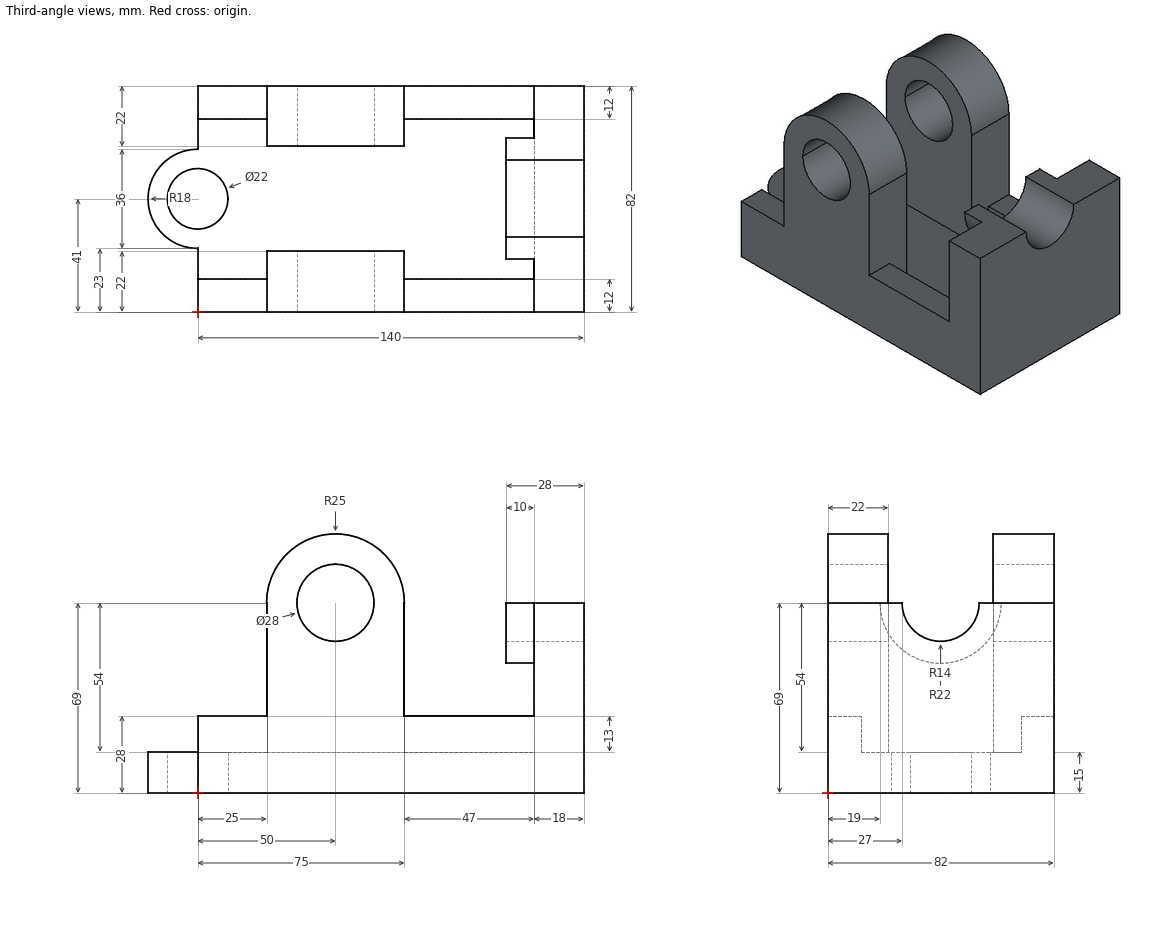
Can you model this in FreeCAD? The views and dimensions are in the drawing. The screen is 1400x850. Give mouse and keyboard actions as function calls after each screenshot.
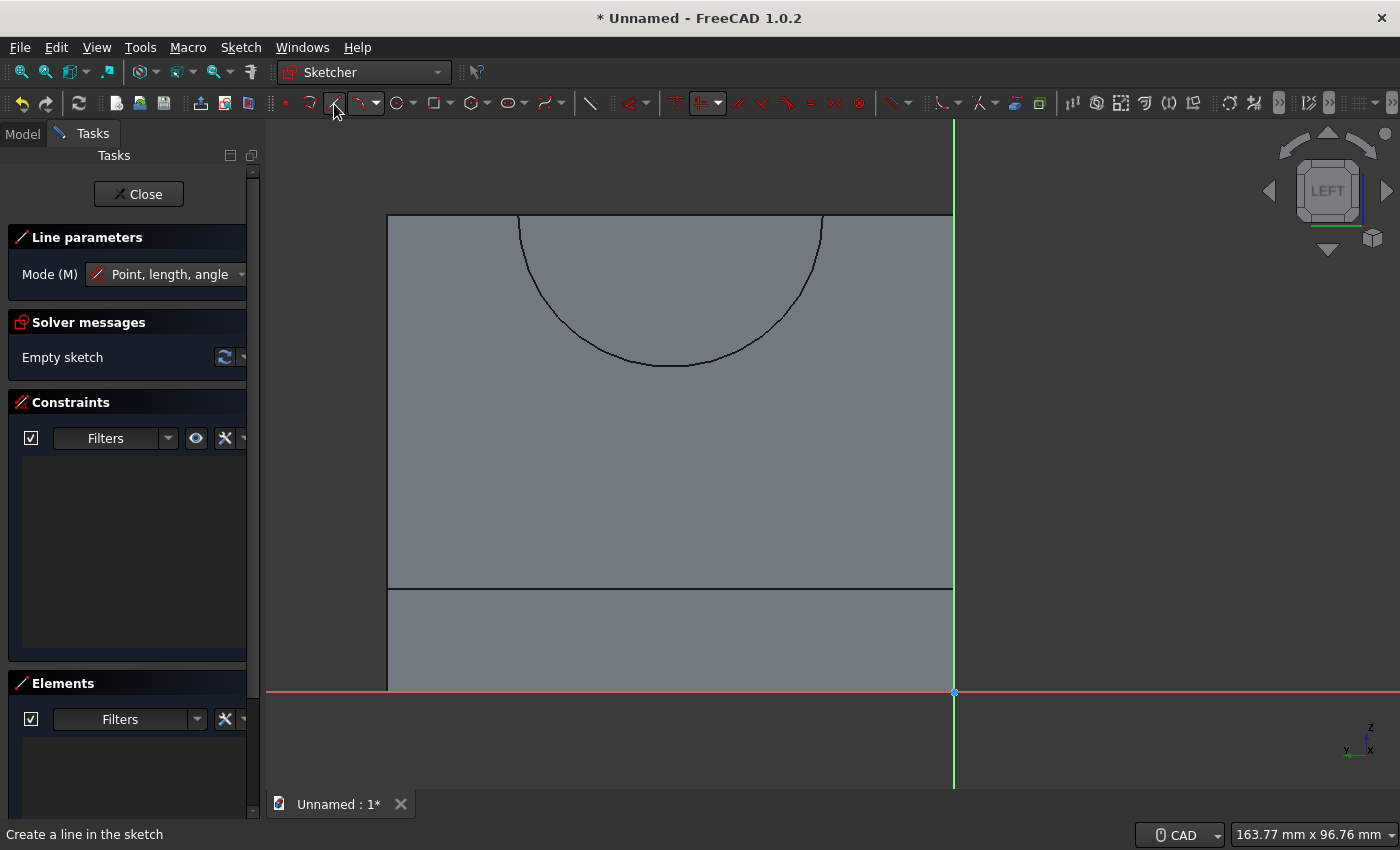
click(767, 215)
click(574, 215)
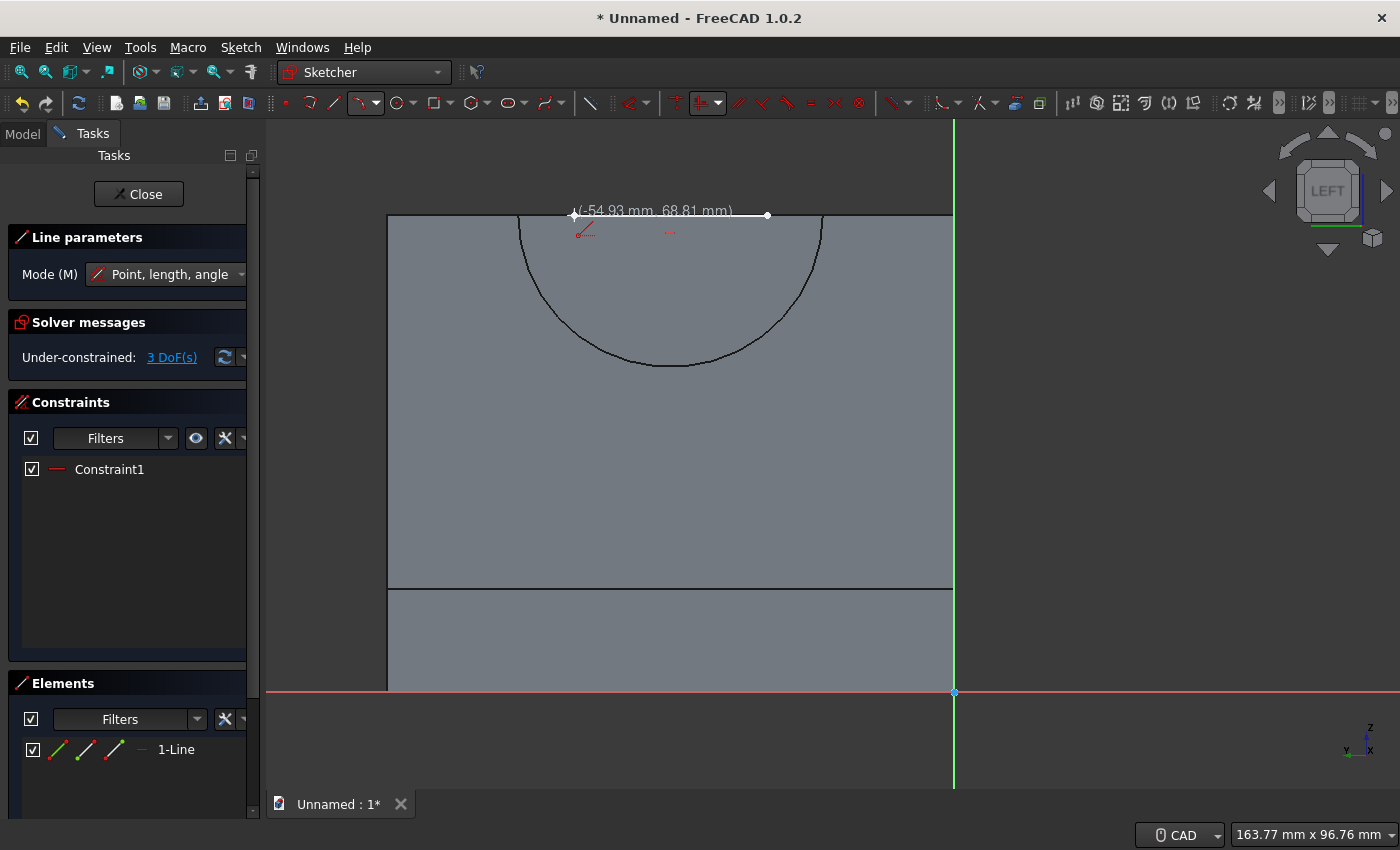
click(360, 104)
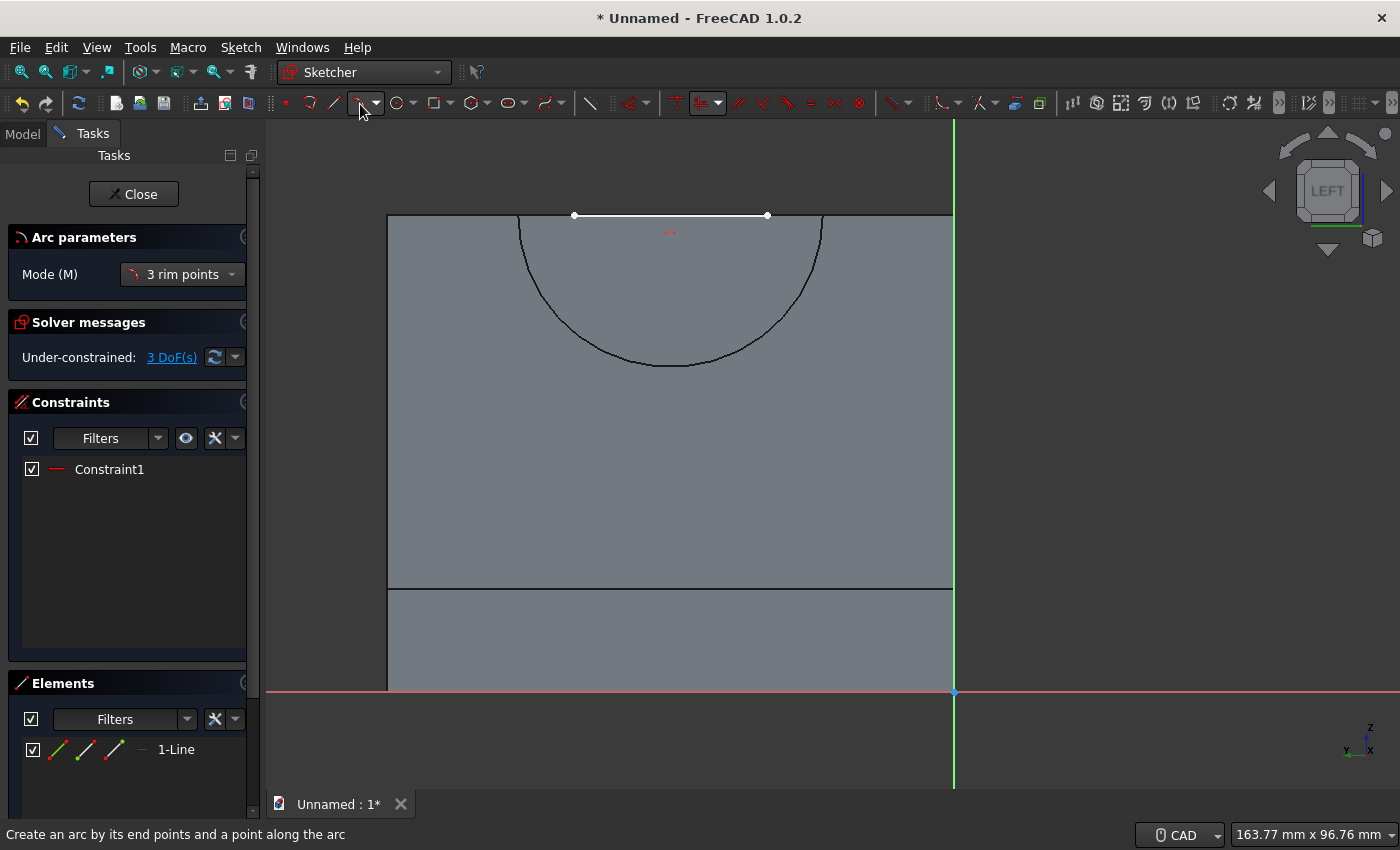
click(574, 216)
click(767, 216)
click(670, 312)
key(Escape)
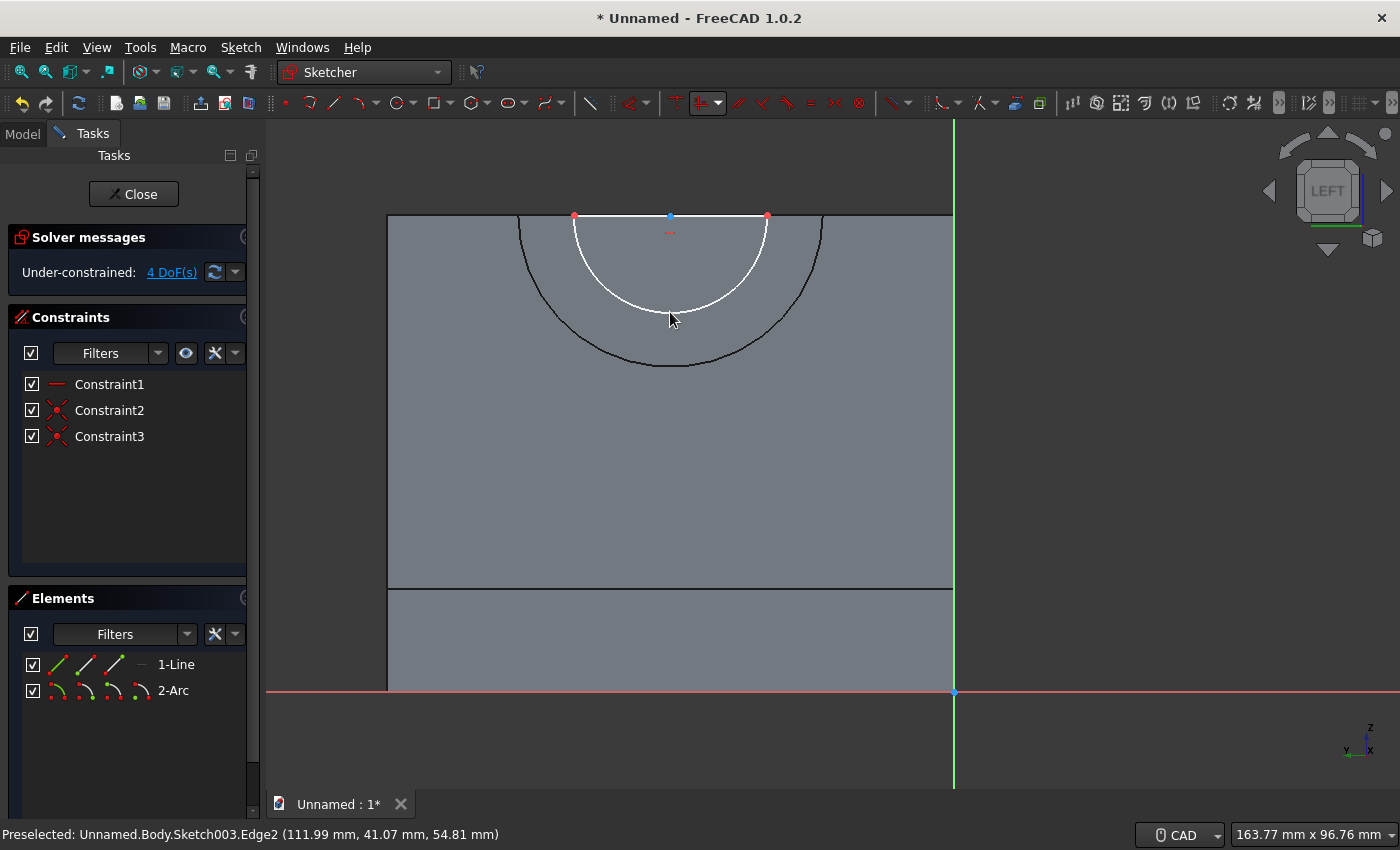
click(630, 104)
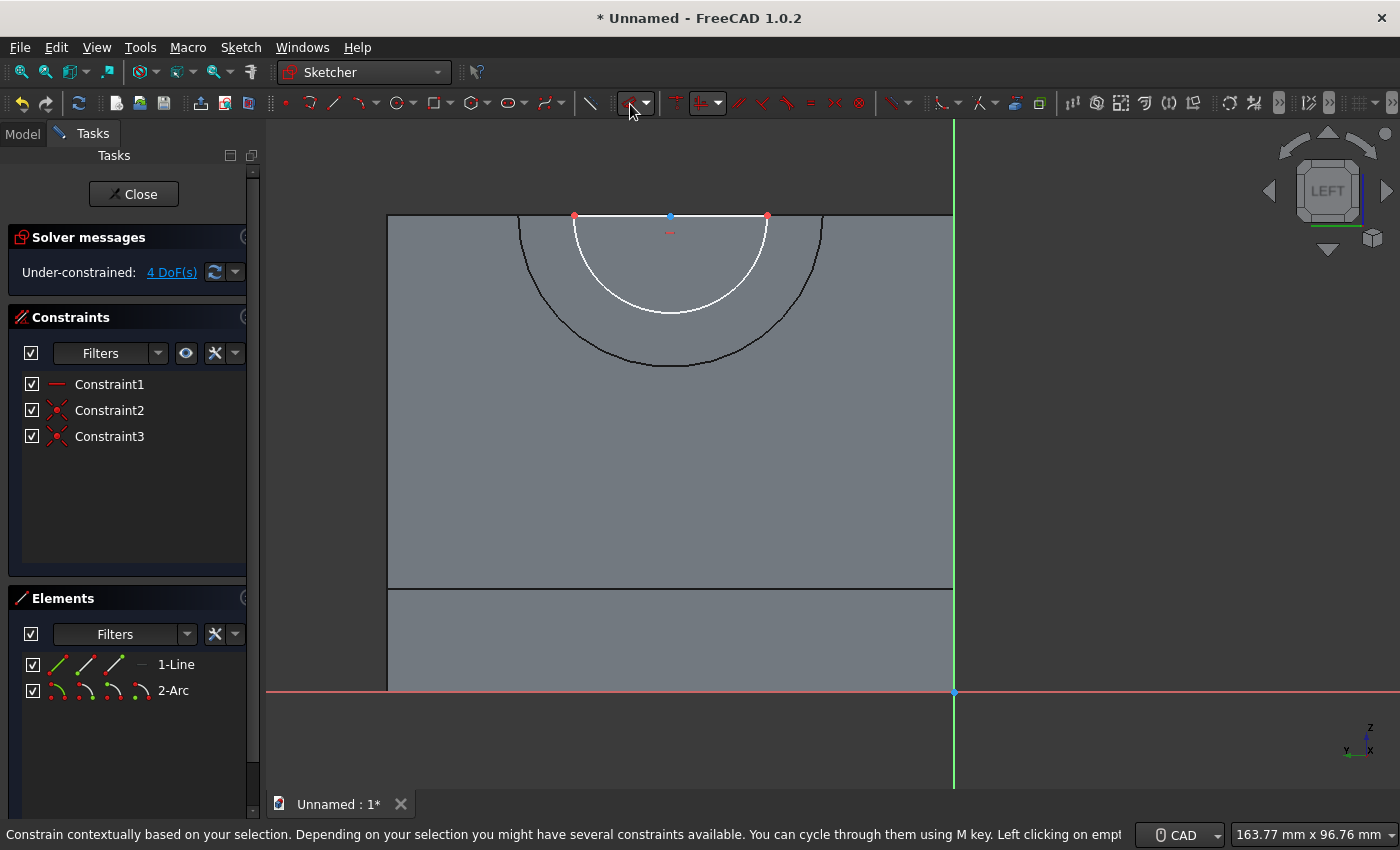
click(614, 294)
click(595, 320)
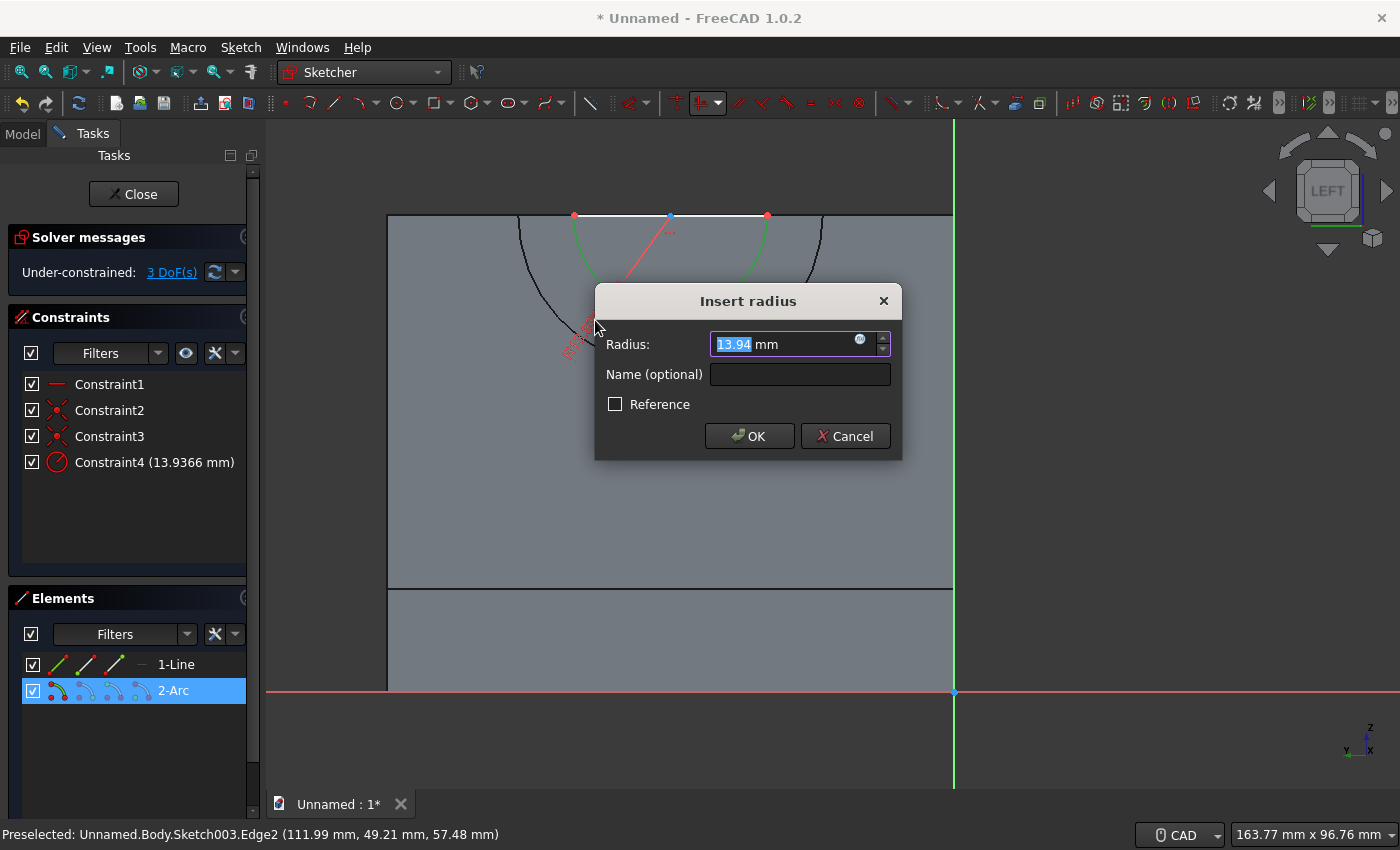
text(14)
key(Return)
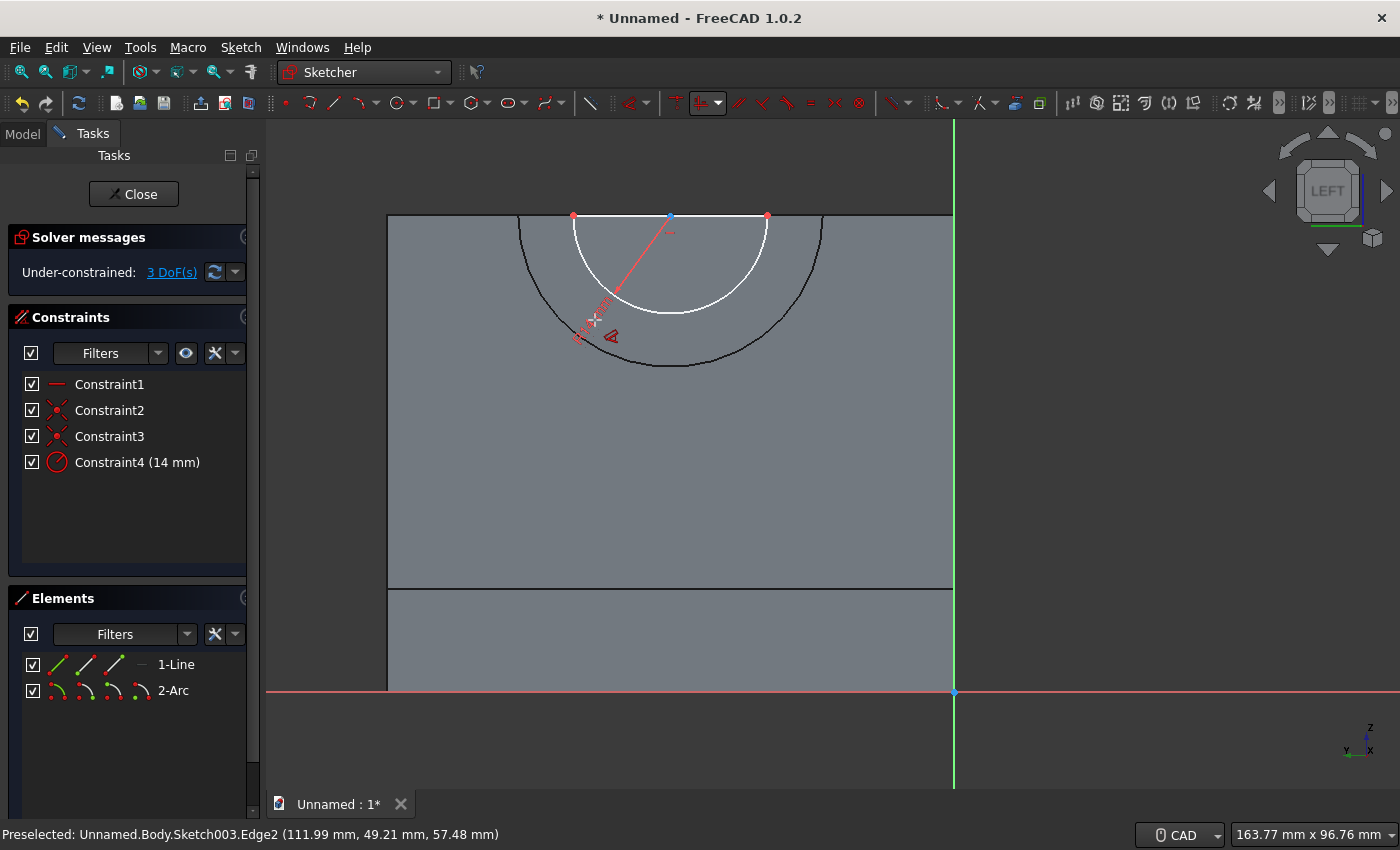
click(767, 216)
click(861, 726)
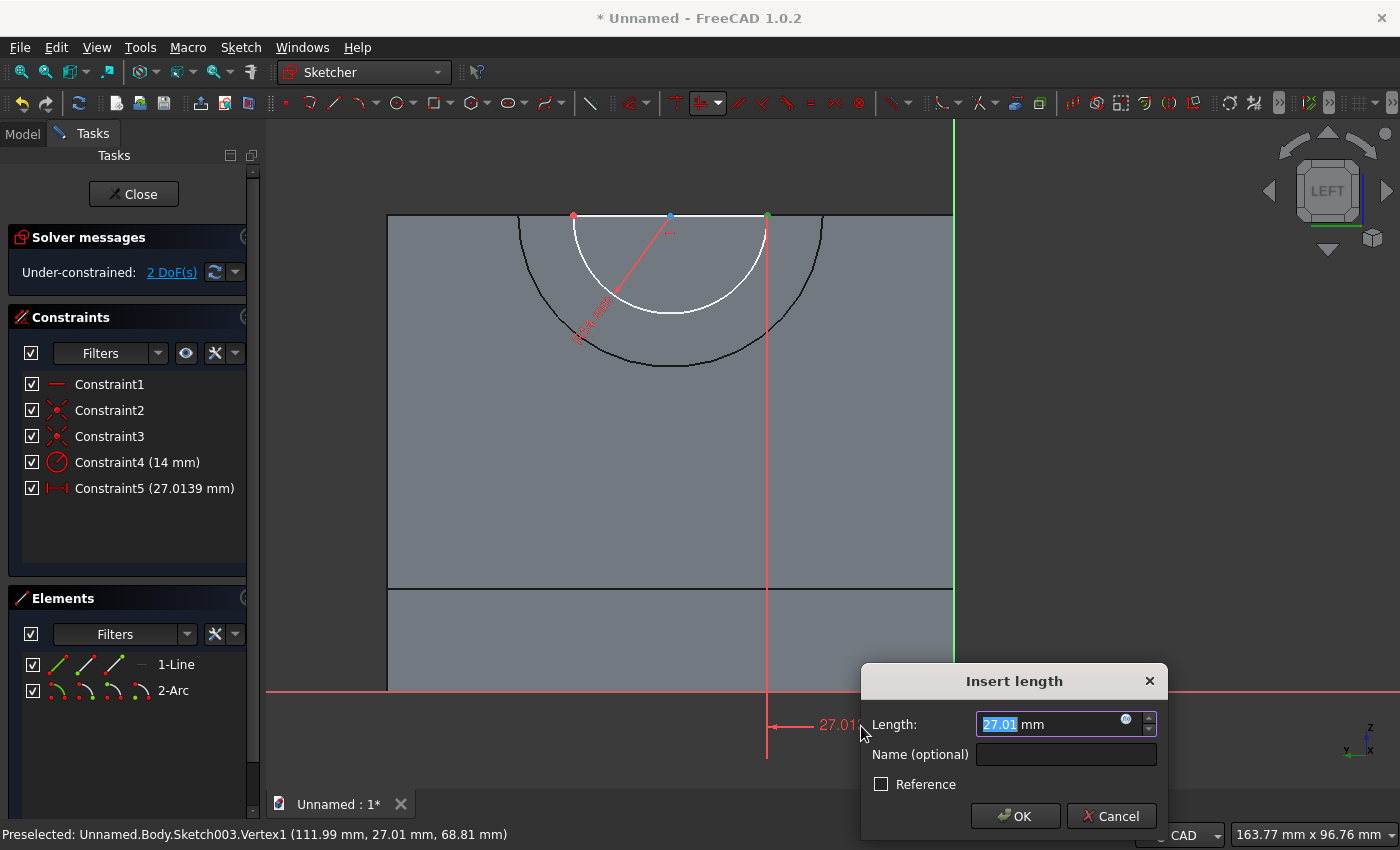
text(27)
key(Return)